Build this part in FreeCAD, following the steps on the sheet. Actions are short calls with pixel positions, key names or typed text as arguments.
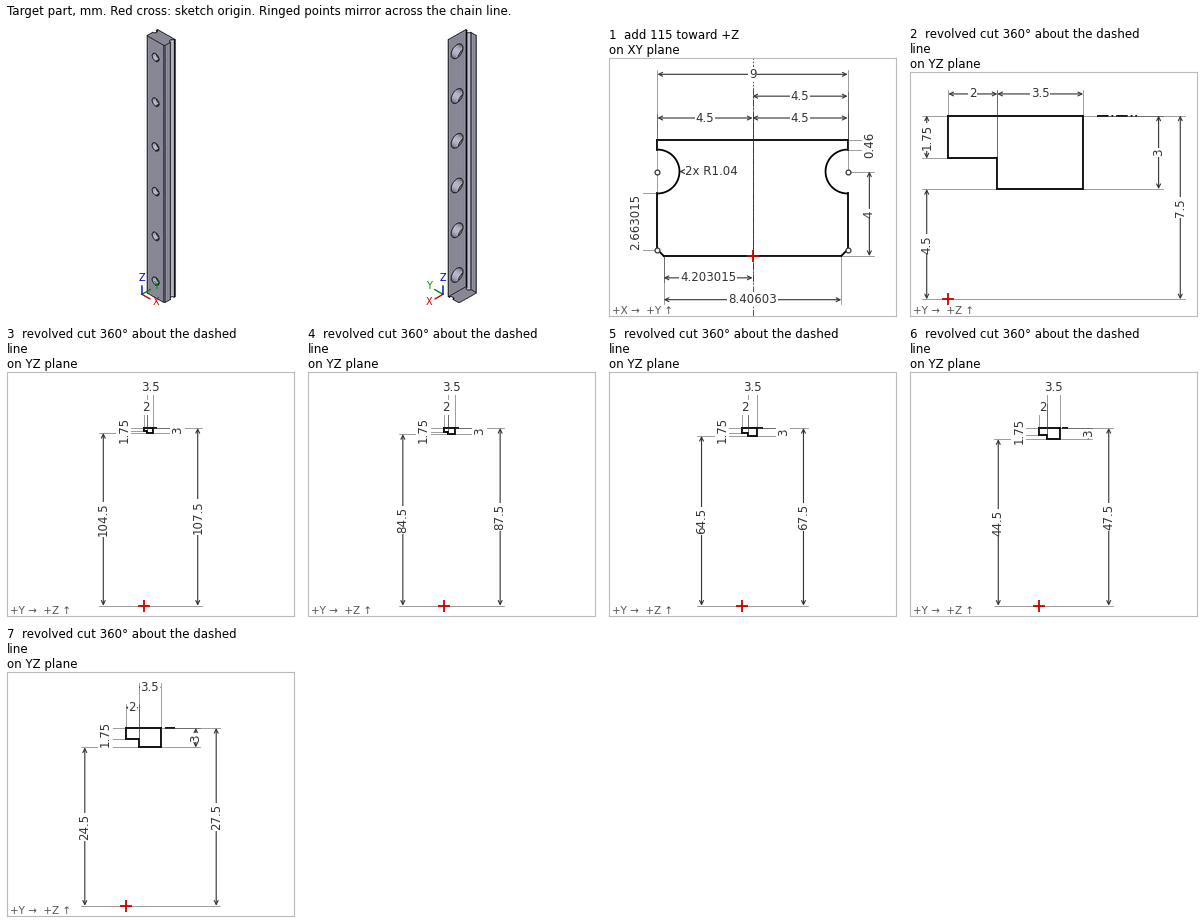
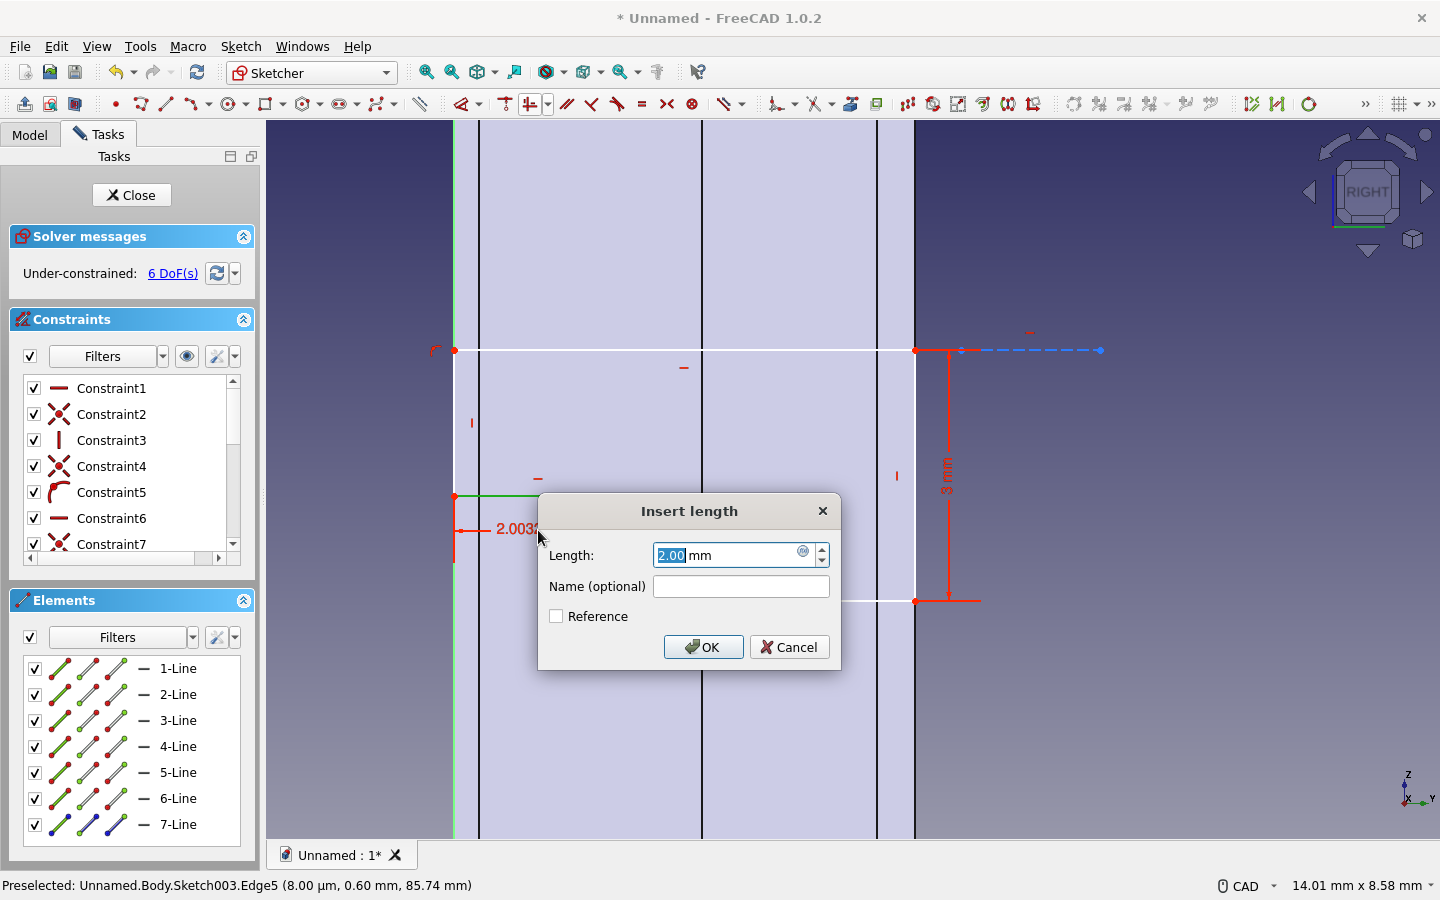
text(2)
key(Return)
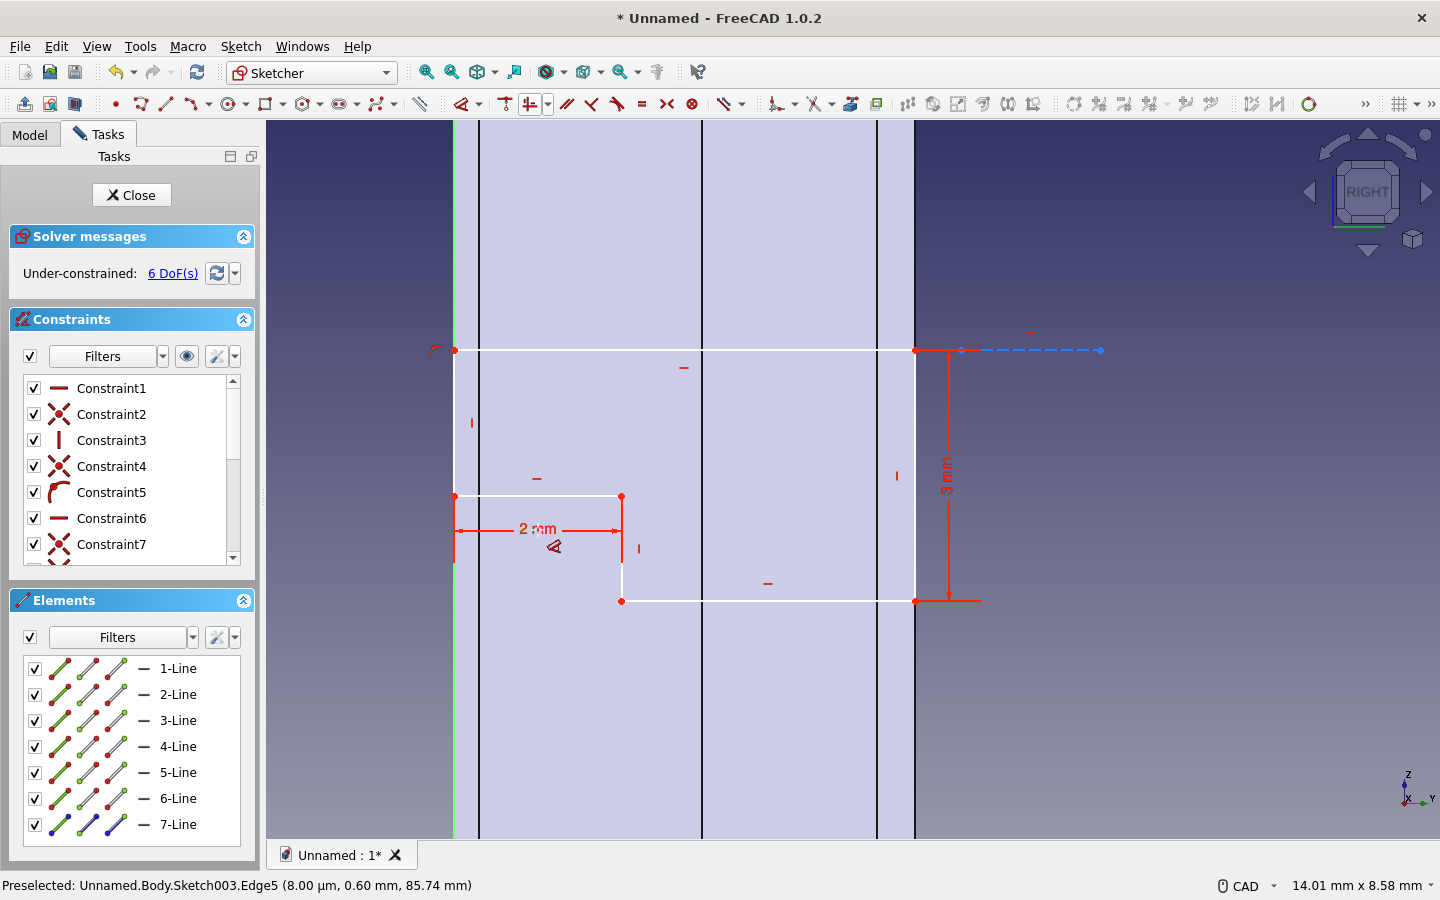
click(710, 601)
click(768, 635)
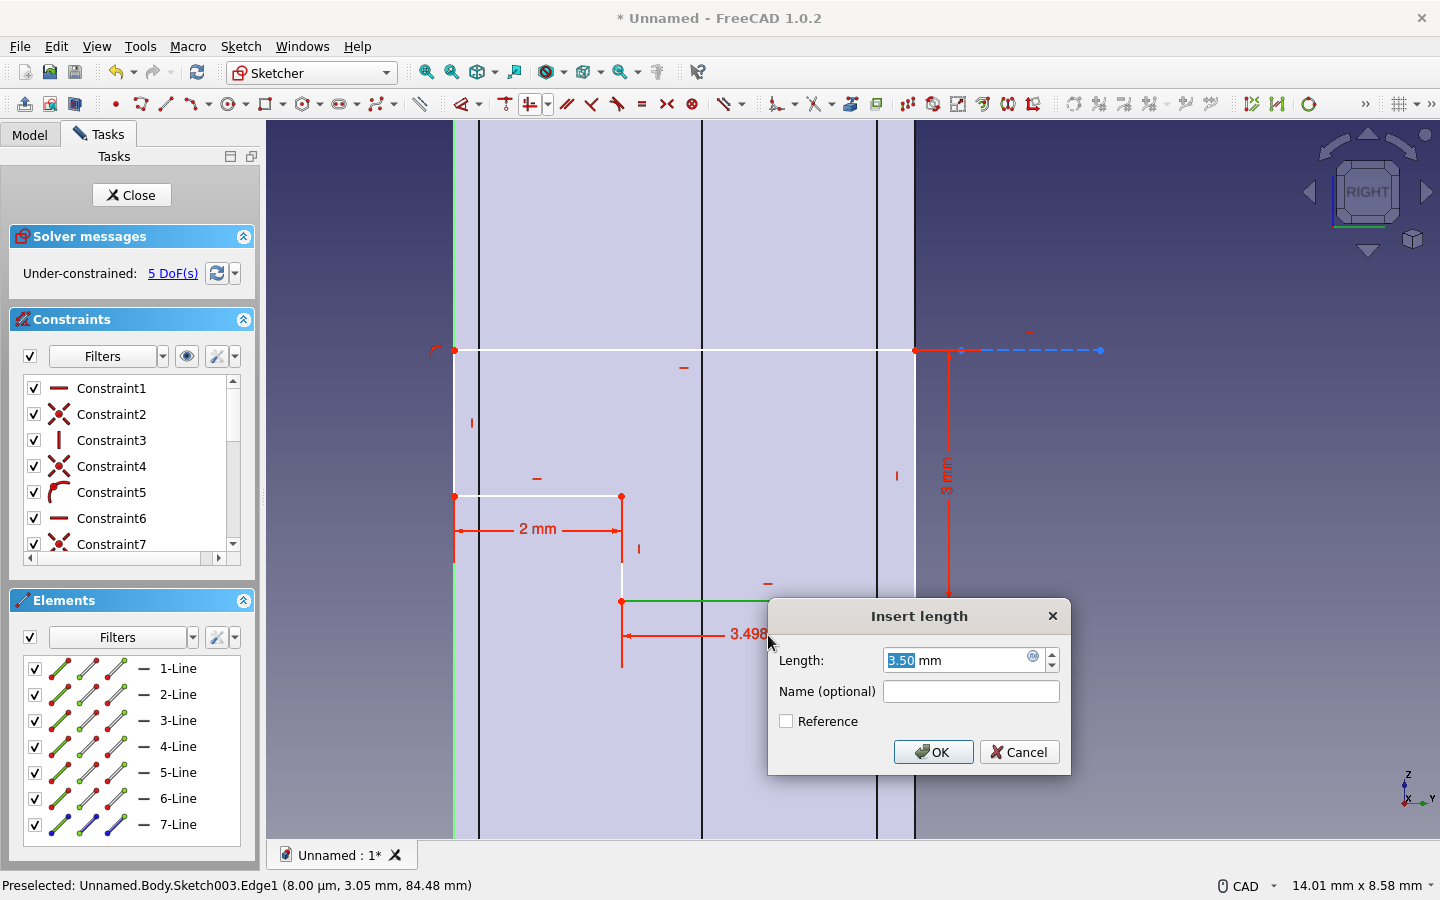
text(3.5)
key(Return)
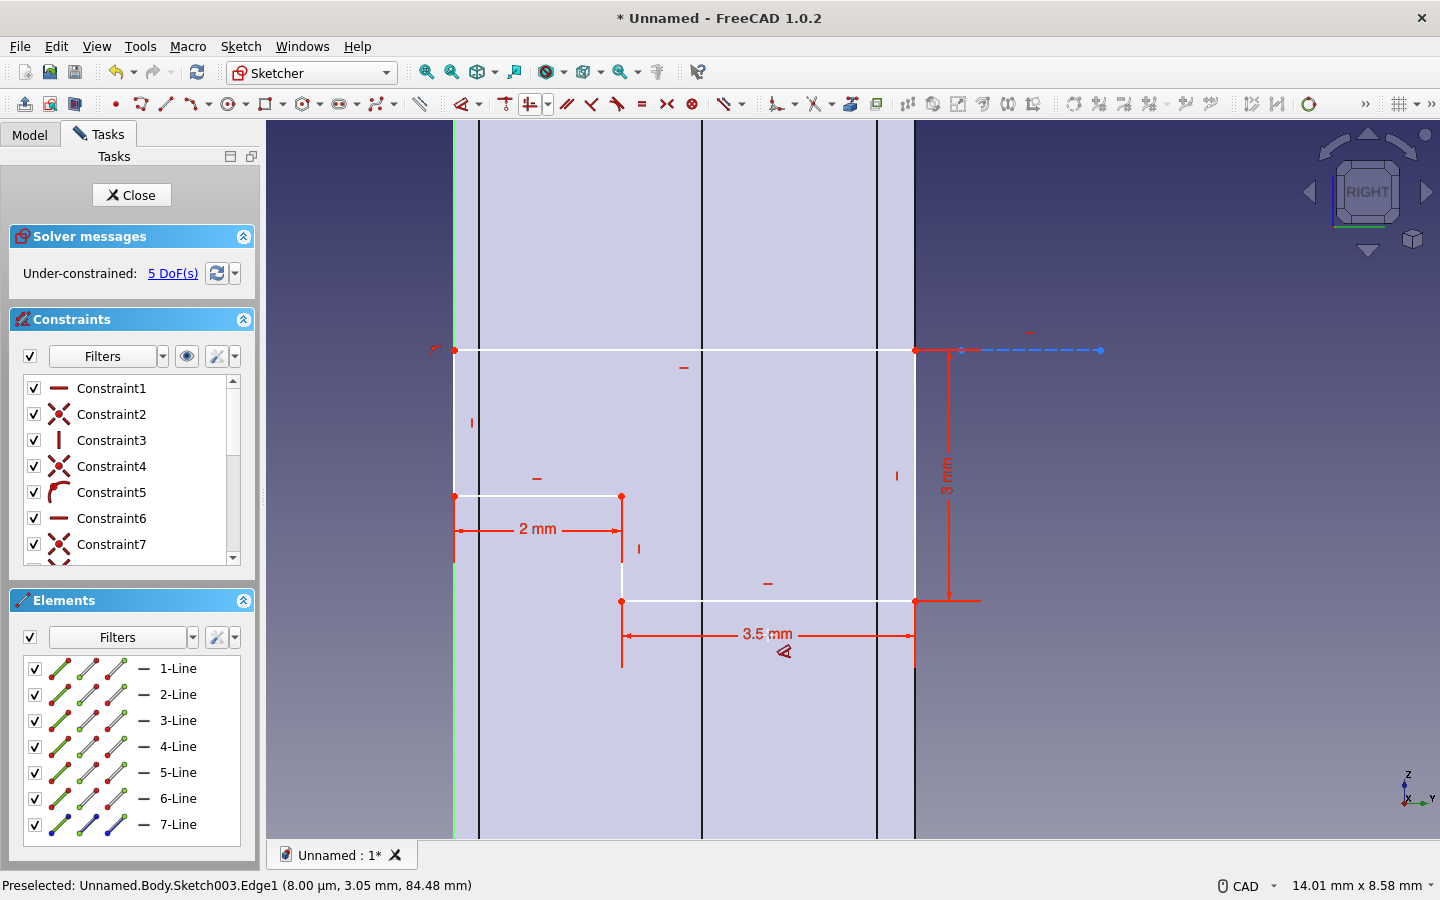
click(454, 394)
click(420, 423)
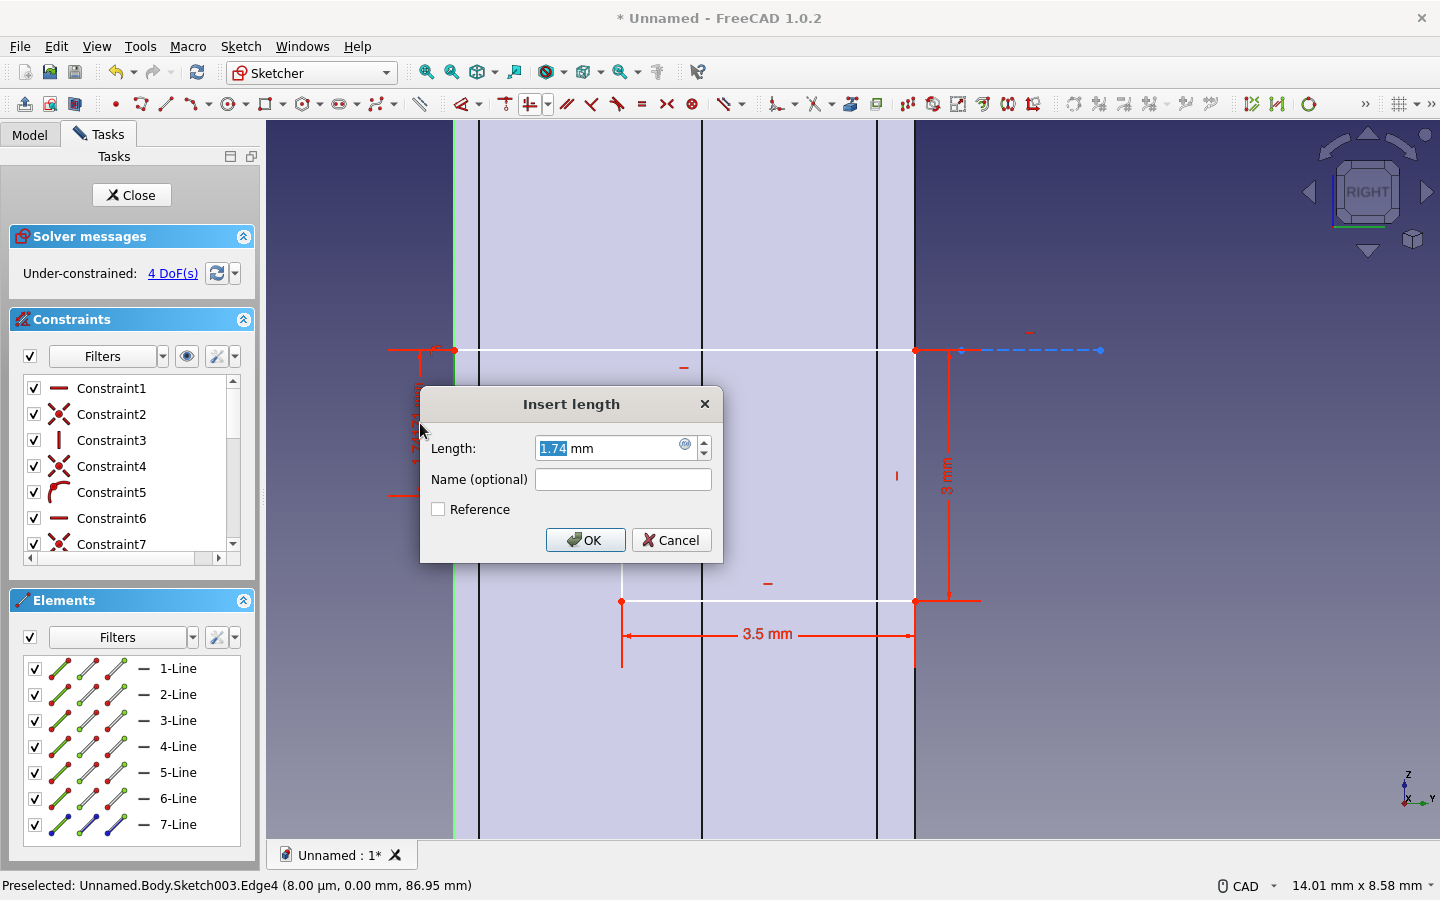
text(1.75)
key(Return)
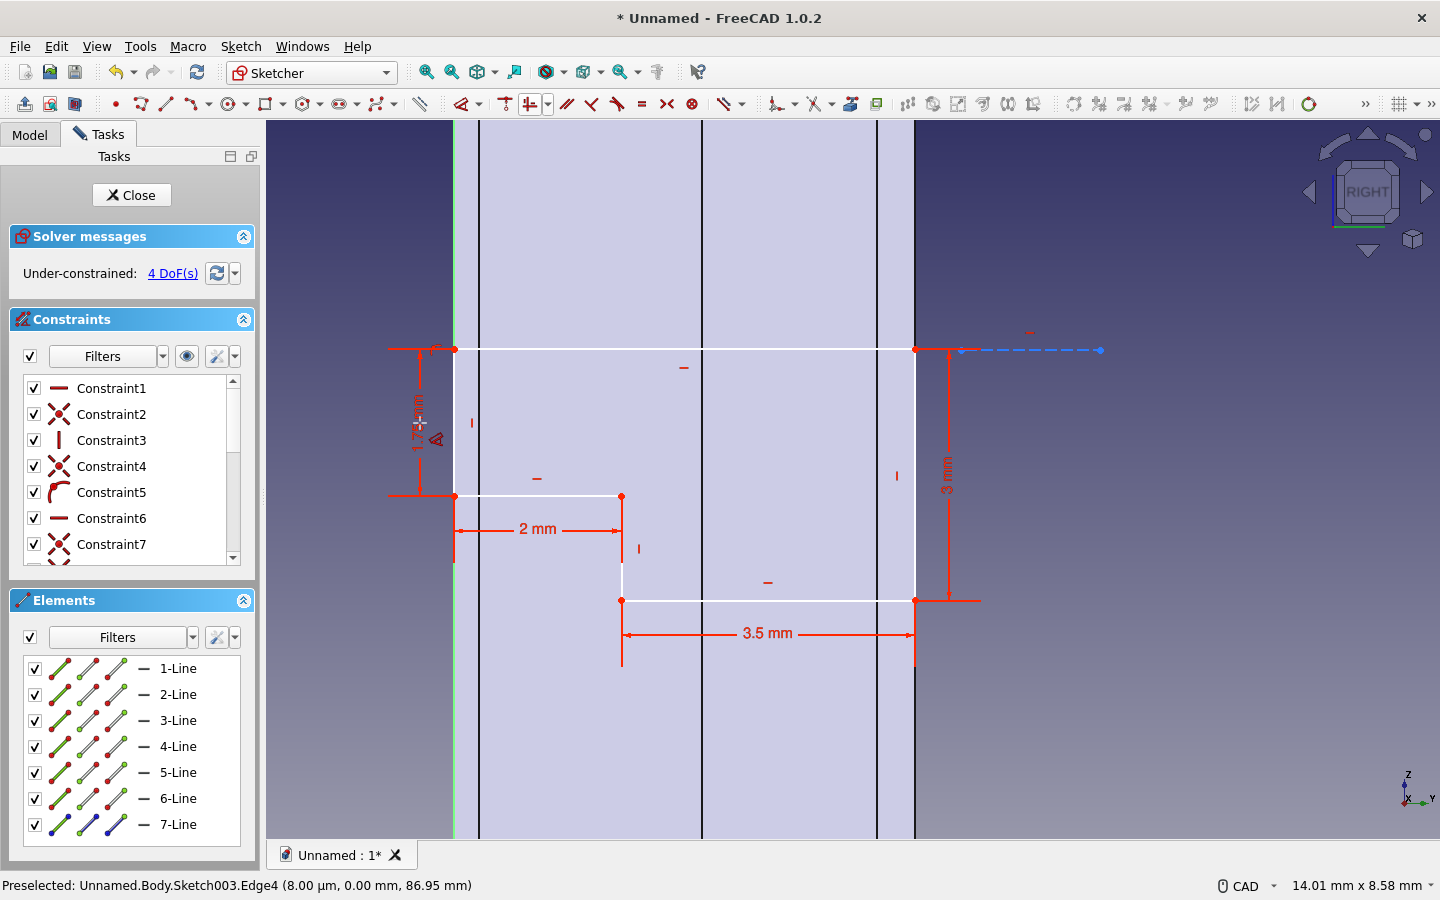
click(622, 601)
click(420, 706)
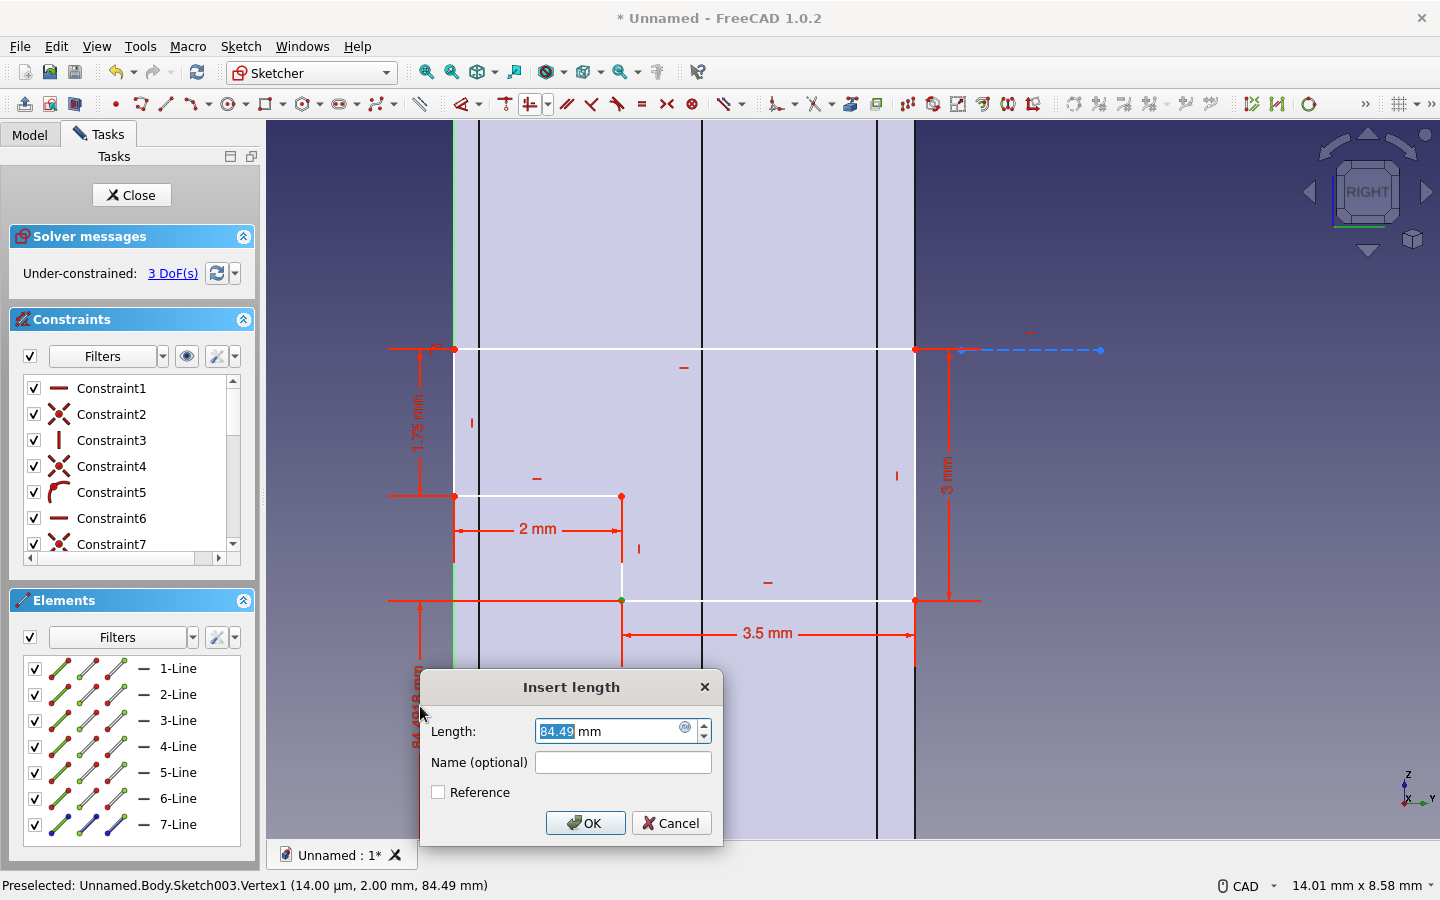
text(84.5)
key(Return)